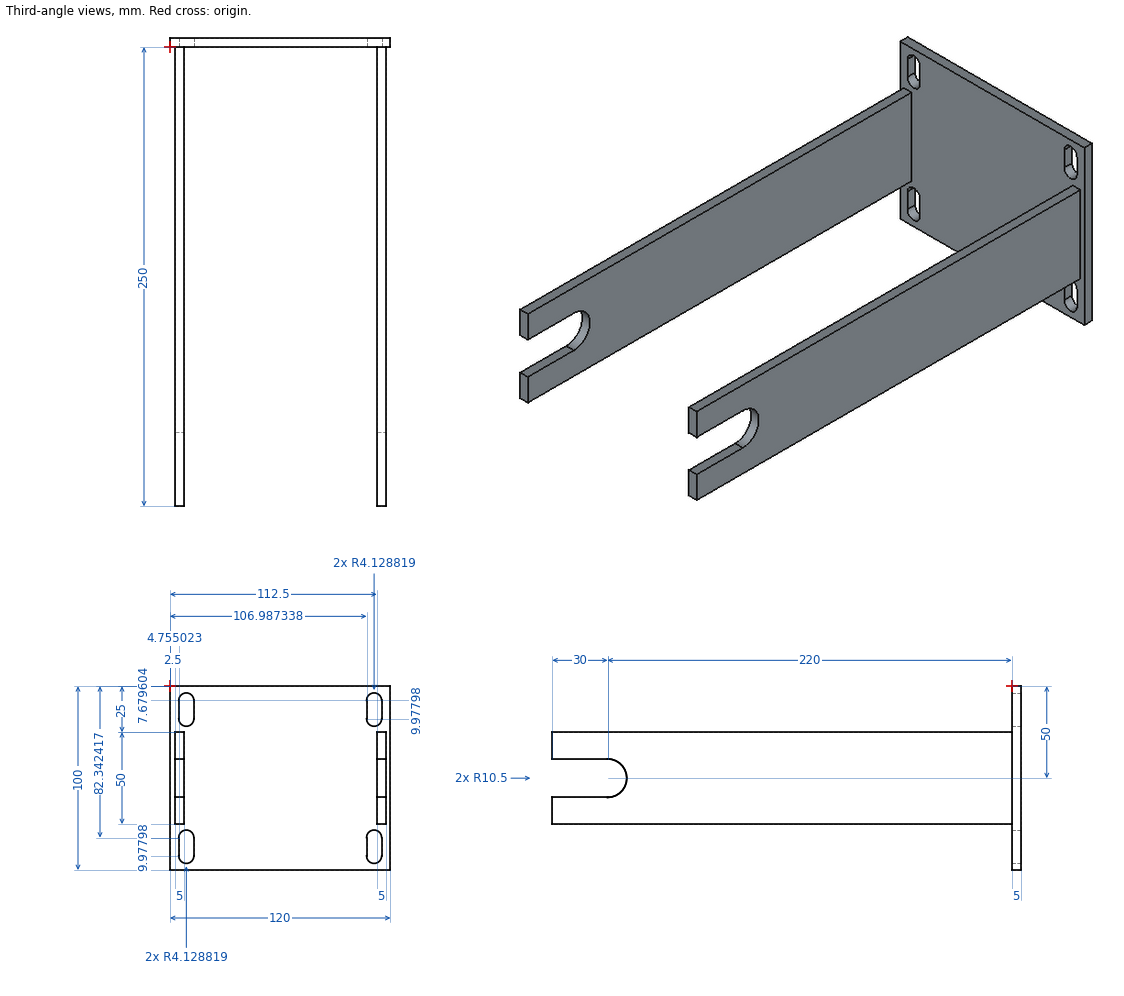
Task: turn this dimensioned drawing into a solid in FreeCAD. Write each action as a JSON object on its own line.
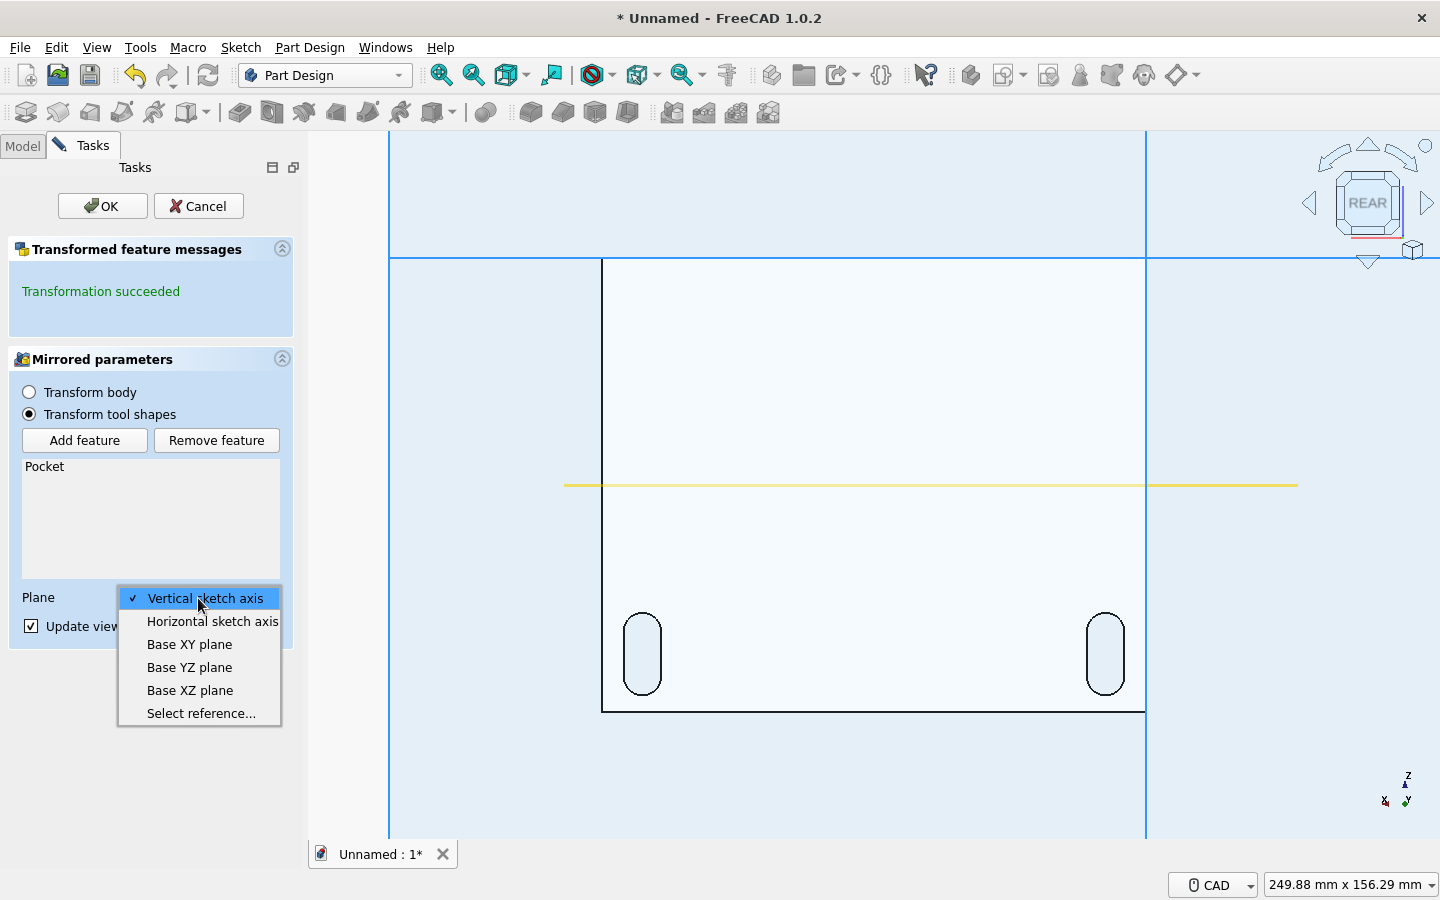
{"action": "left_click", "coordinate": [198, 714]}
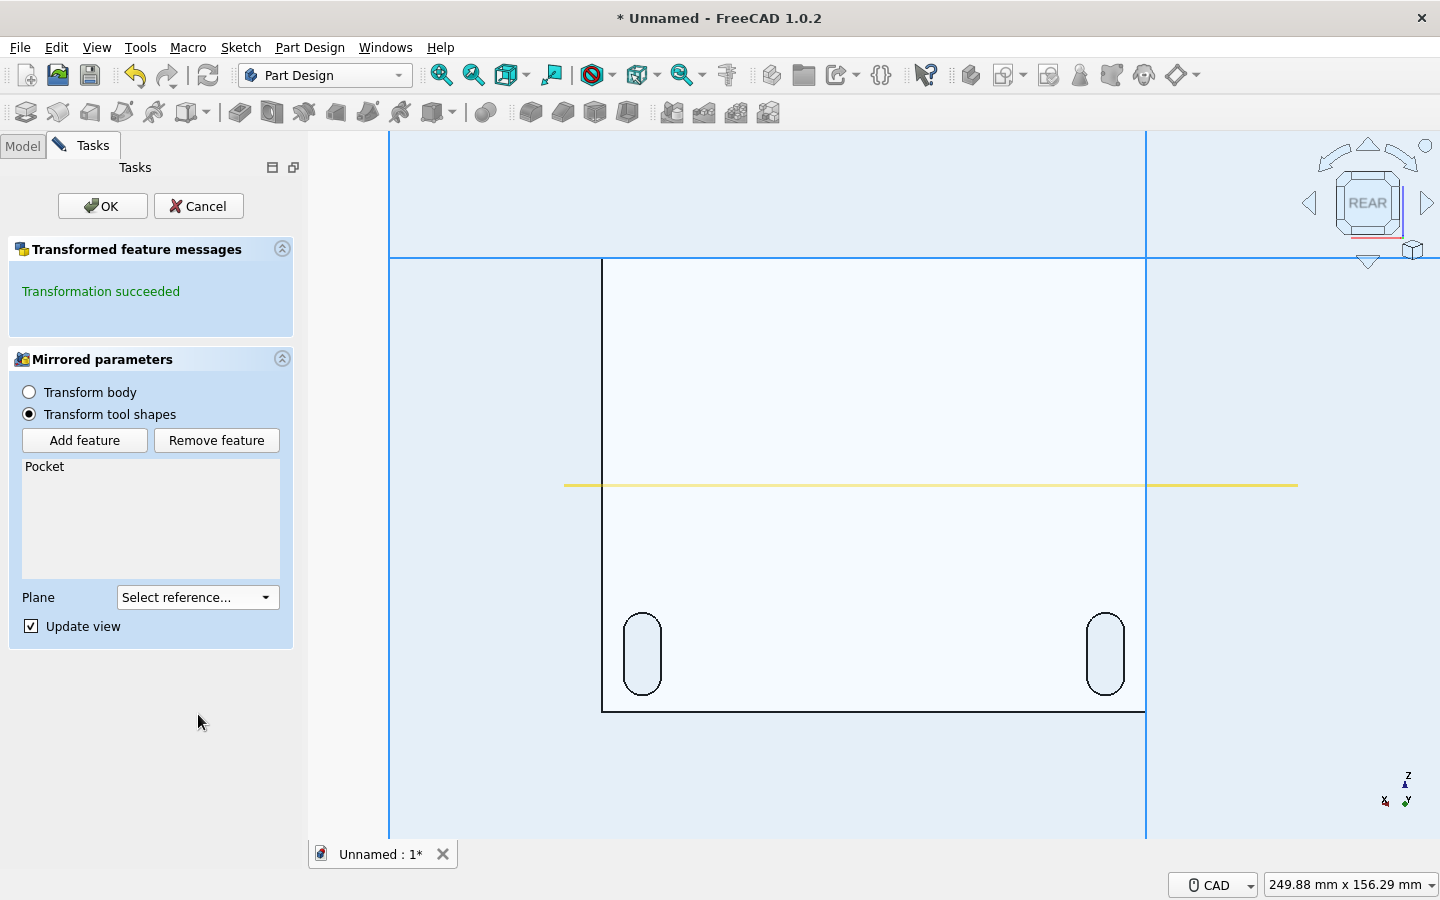
{"action": "left_click", "coordinate": [23, 145]}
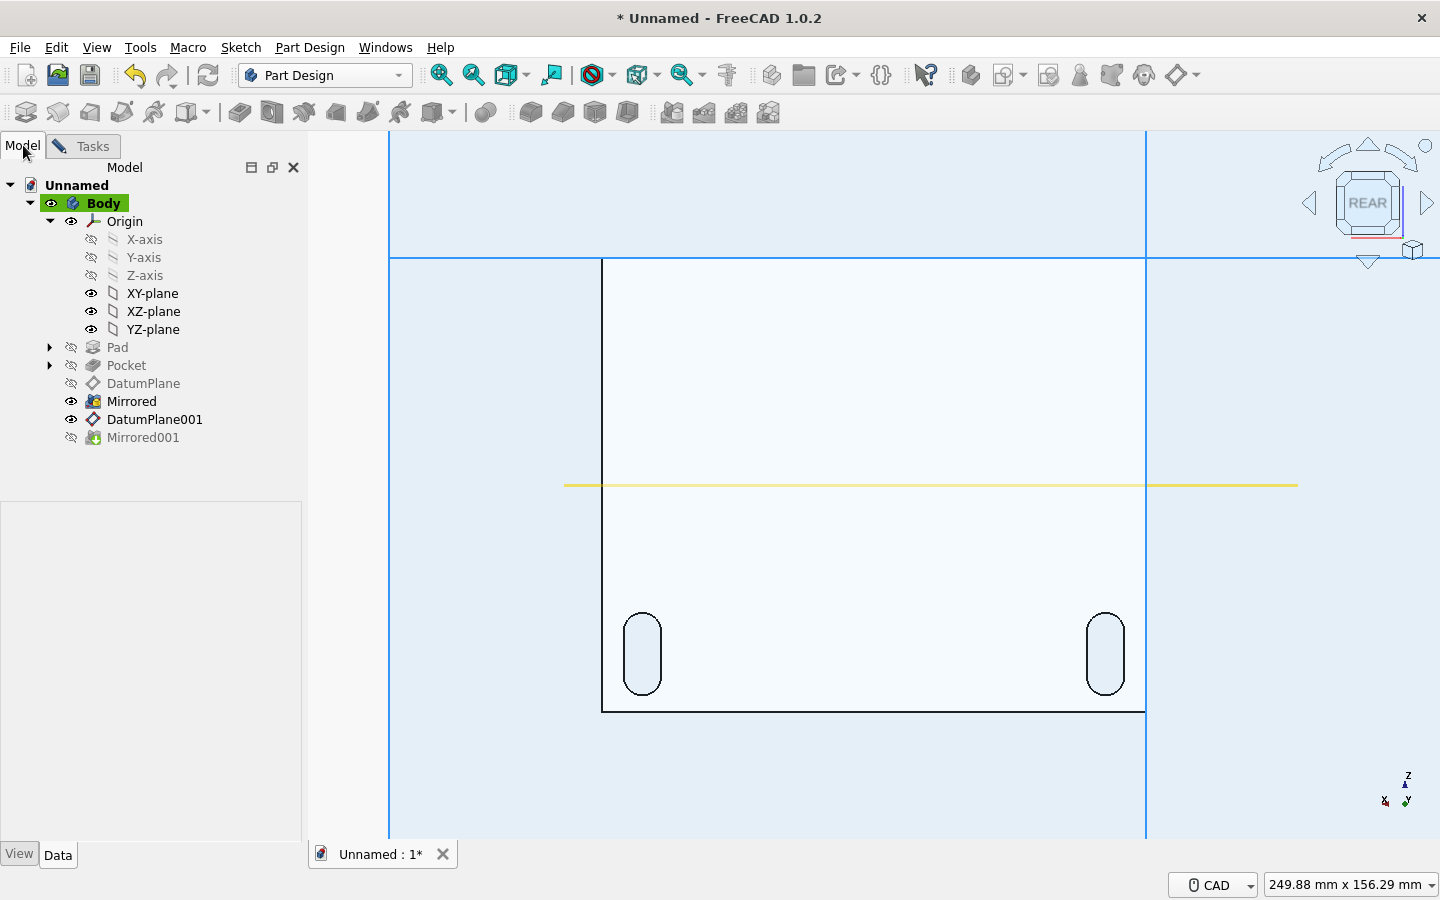
{"action": "left_click", "coordinate": [116, 419]}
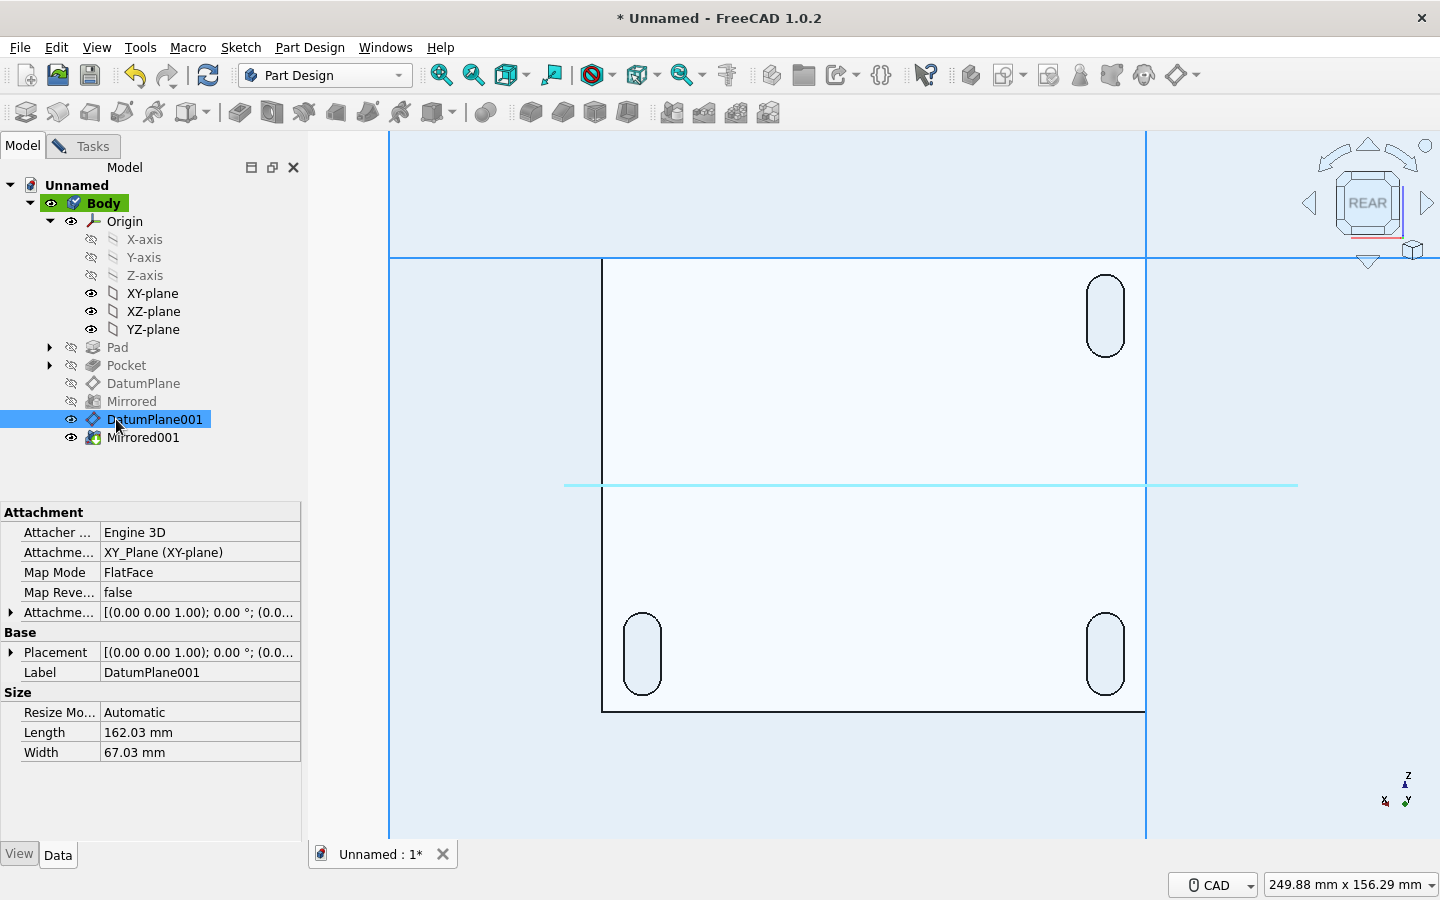
{"action": "left_click", "coordinate": [84, 145]}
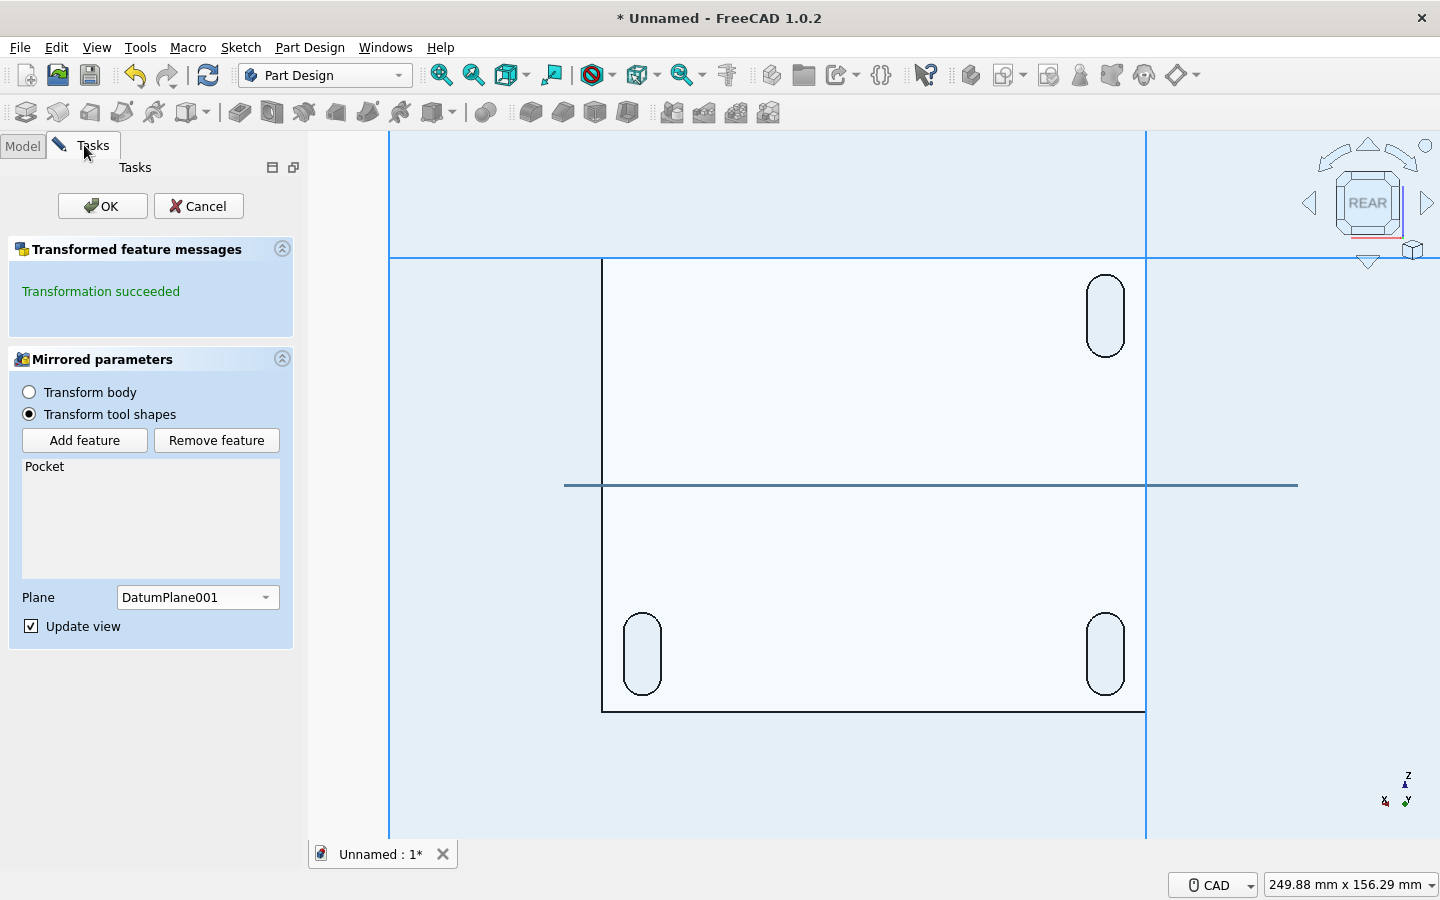
{"action": "left_click", "coordinate": [103, 206]}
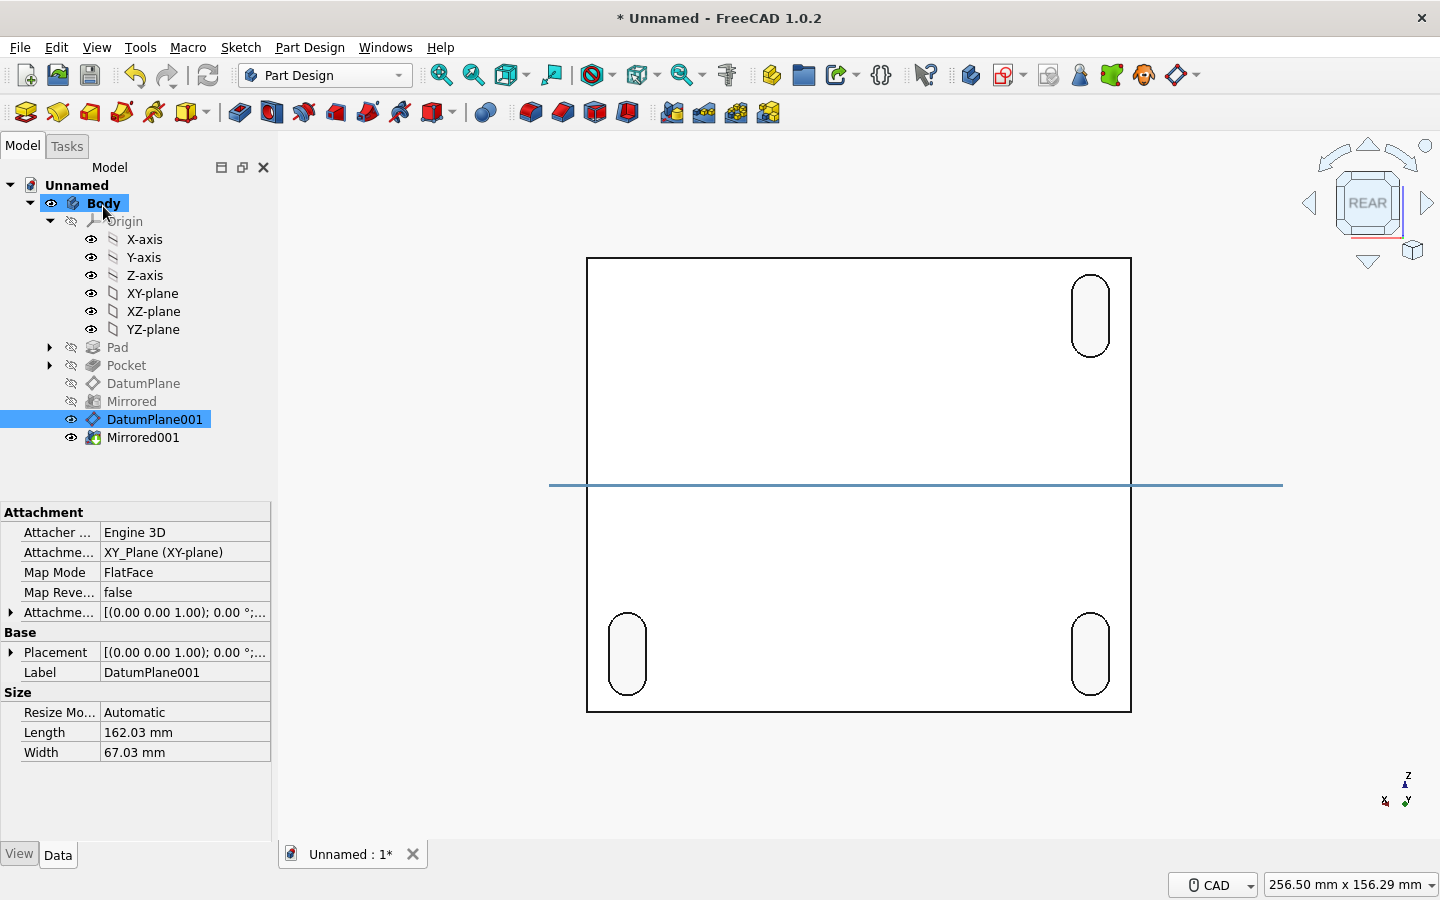
{"action": "left_click", "coordinate": [116, 419]}
{"action": "key", "text": "space"}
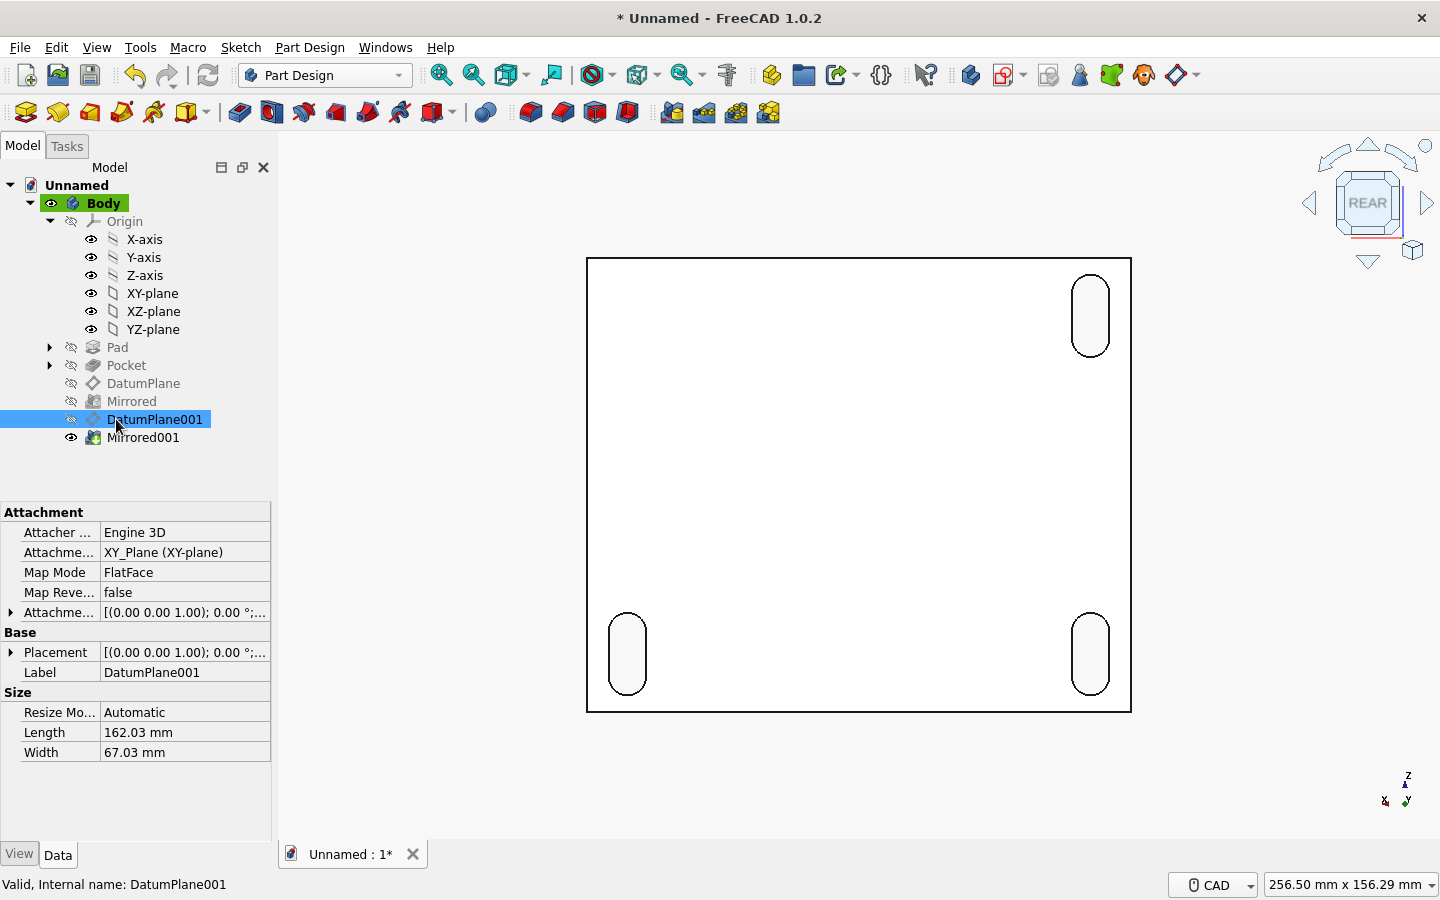
{"action": "left_click", "coordinate": [859, 484]}